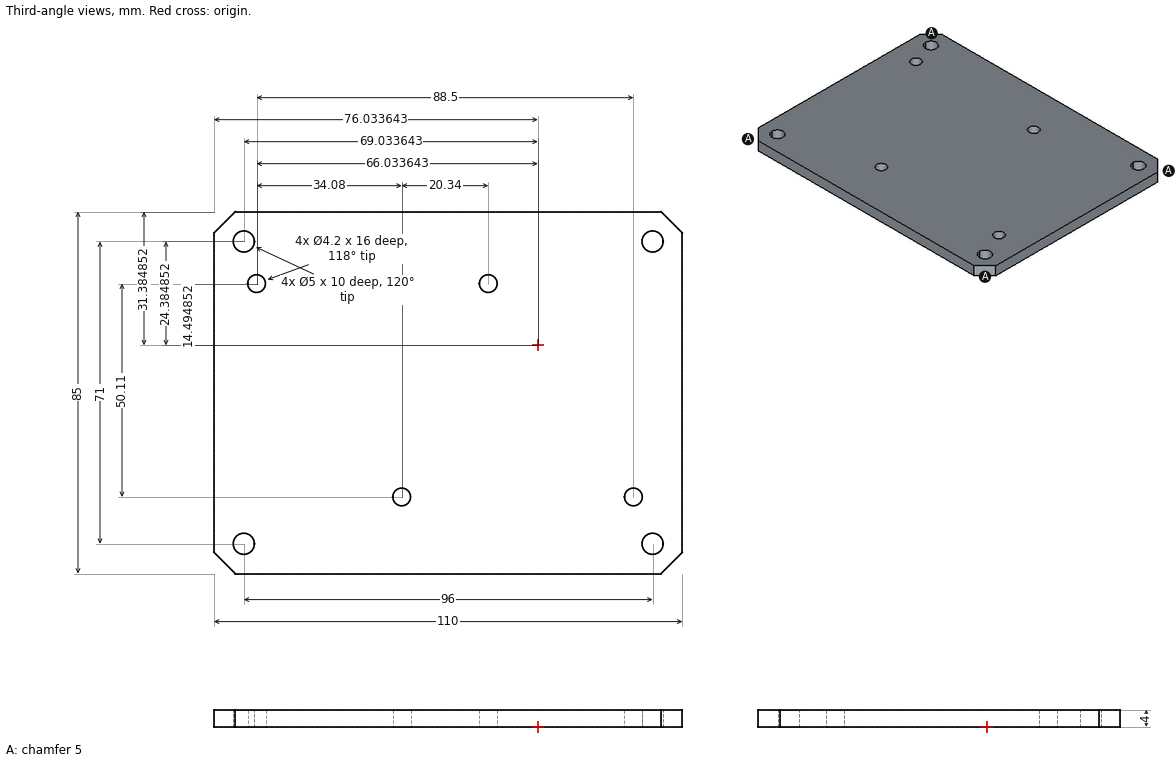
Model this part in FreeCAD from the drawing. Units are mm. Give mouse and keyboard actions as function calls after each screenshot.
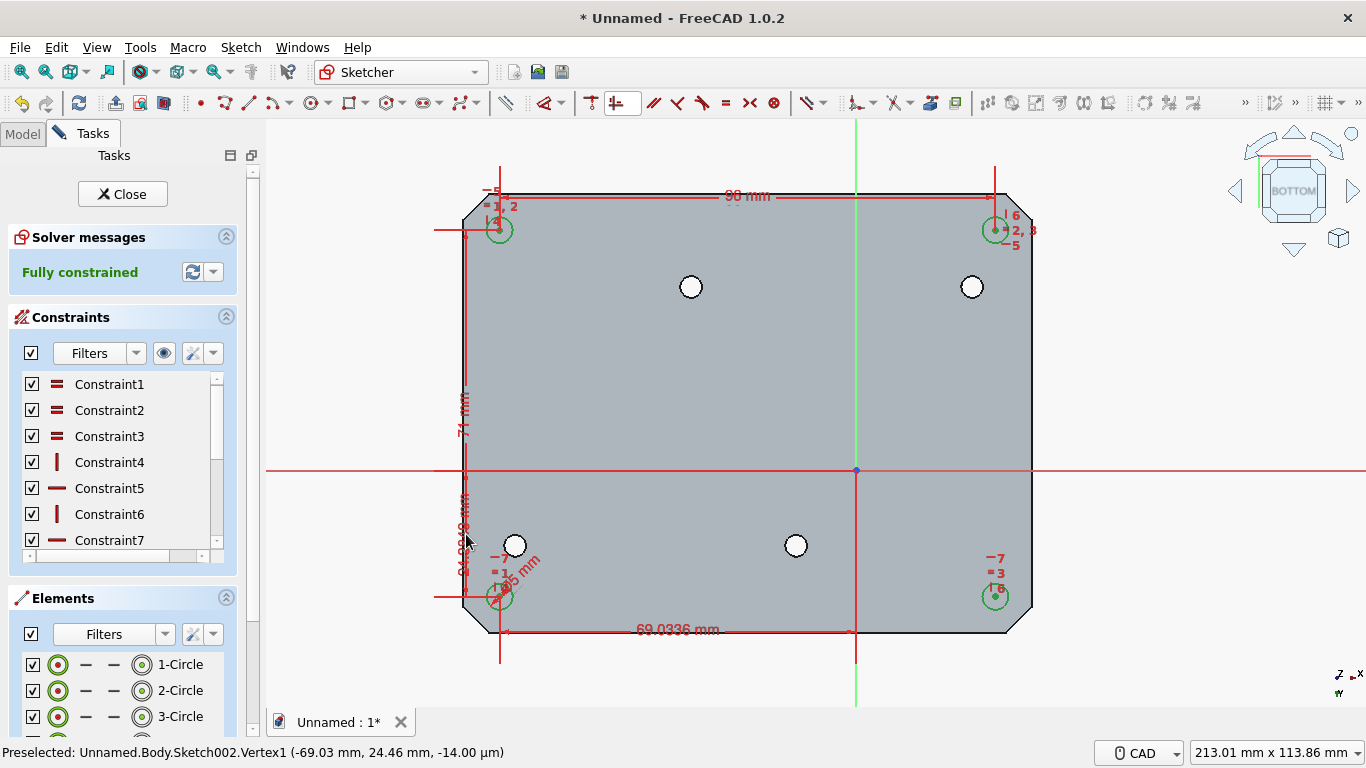
click(123, 194)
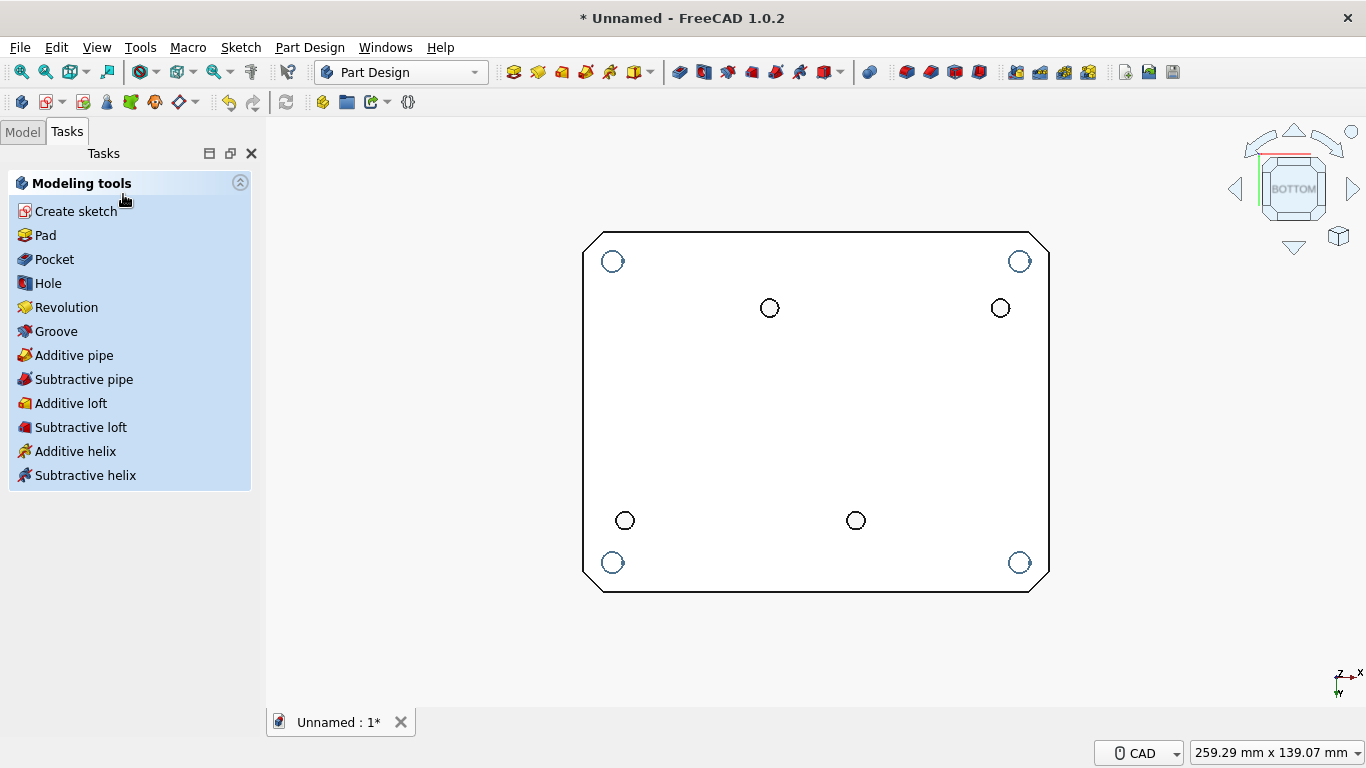
click(704, 72)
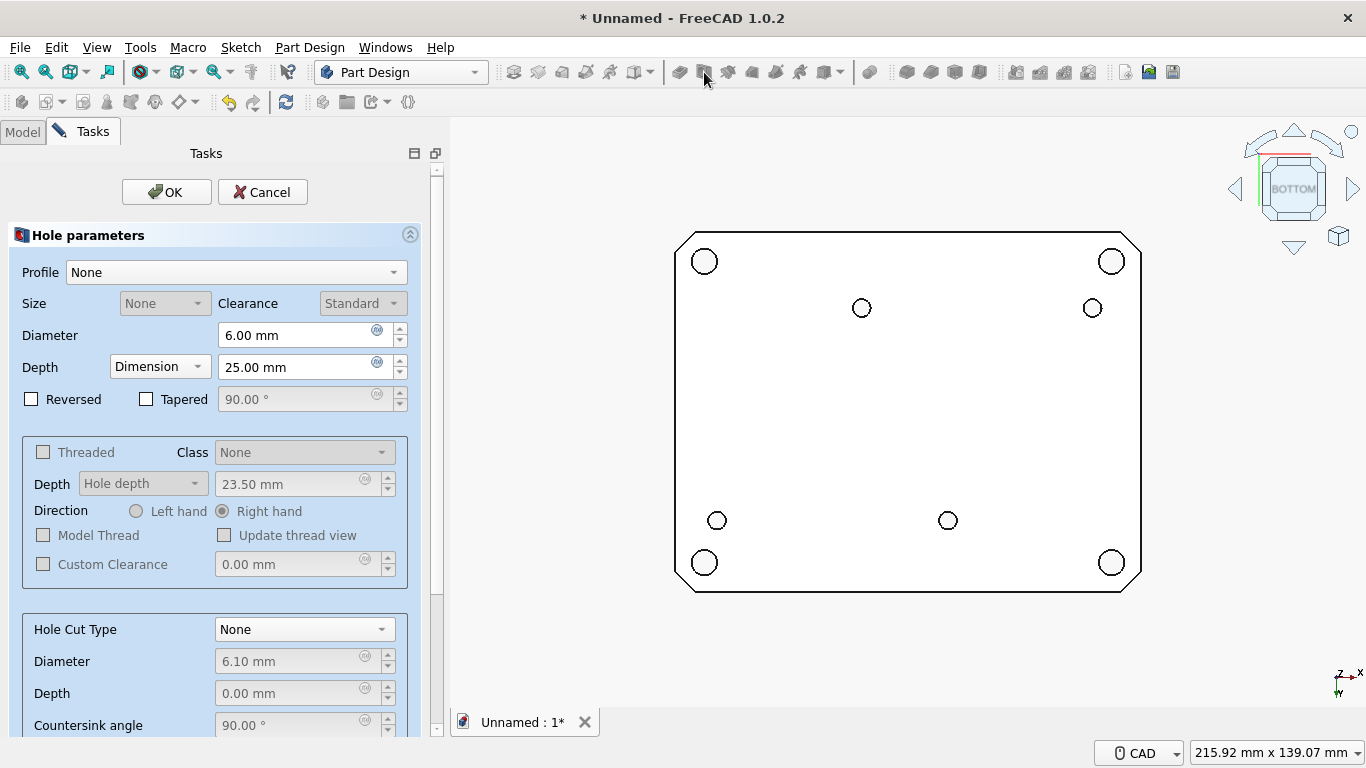
triple_click(305, 335)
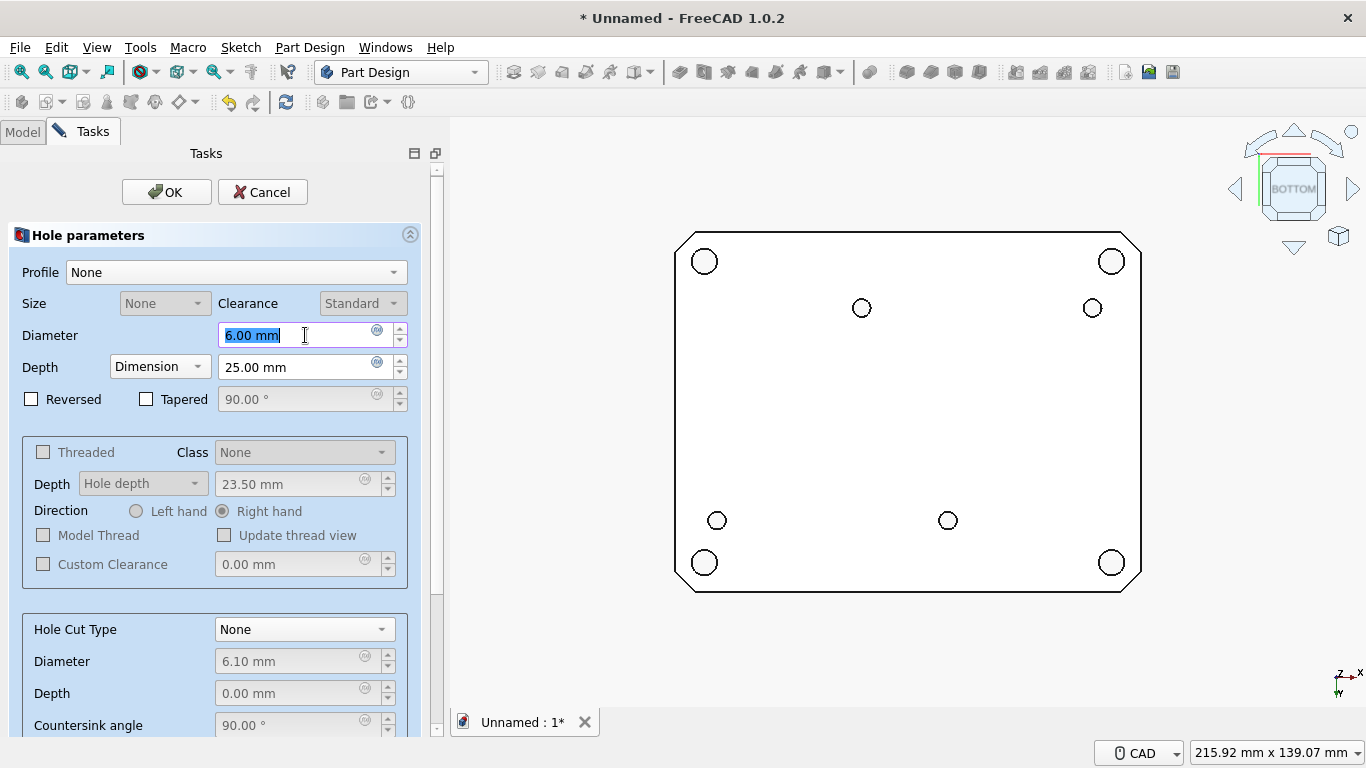
text(5)
key(Tab)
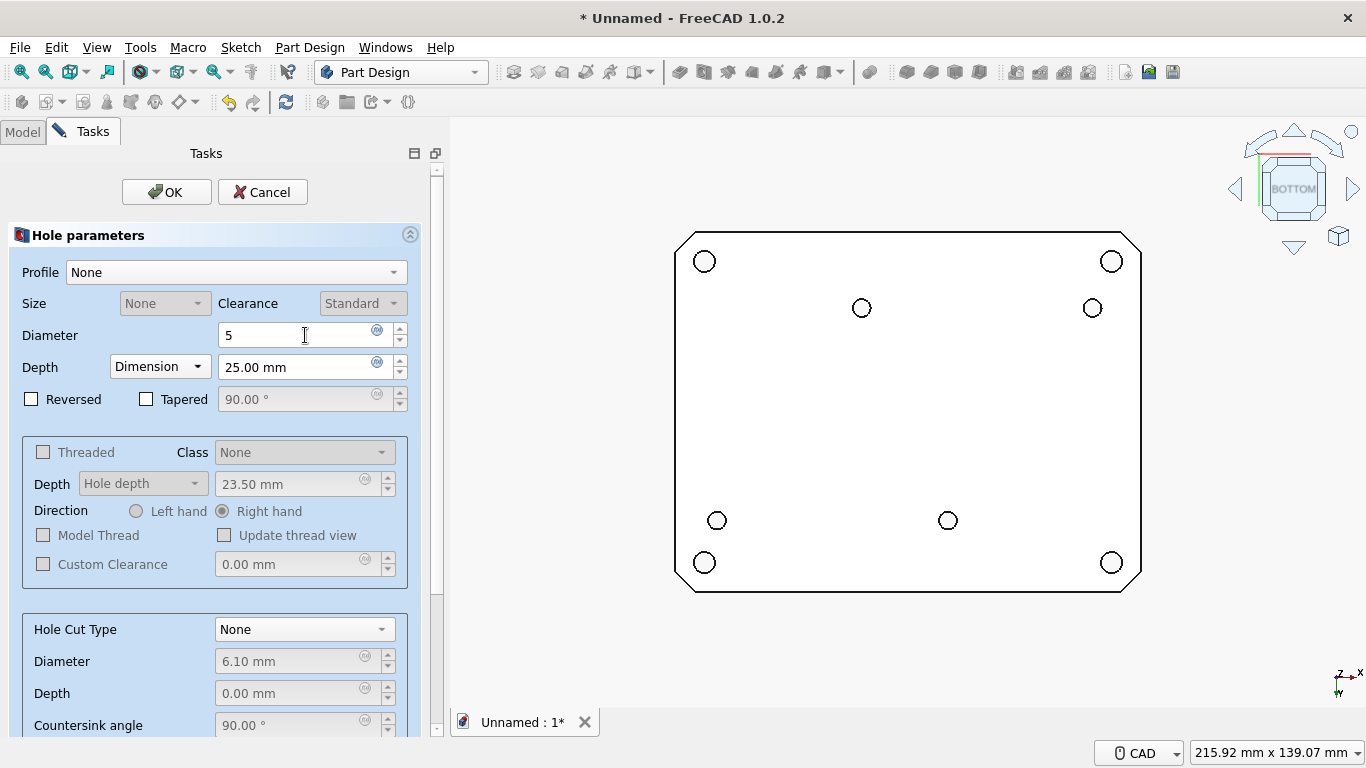
triple_click(305, 367)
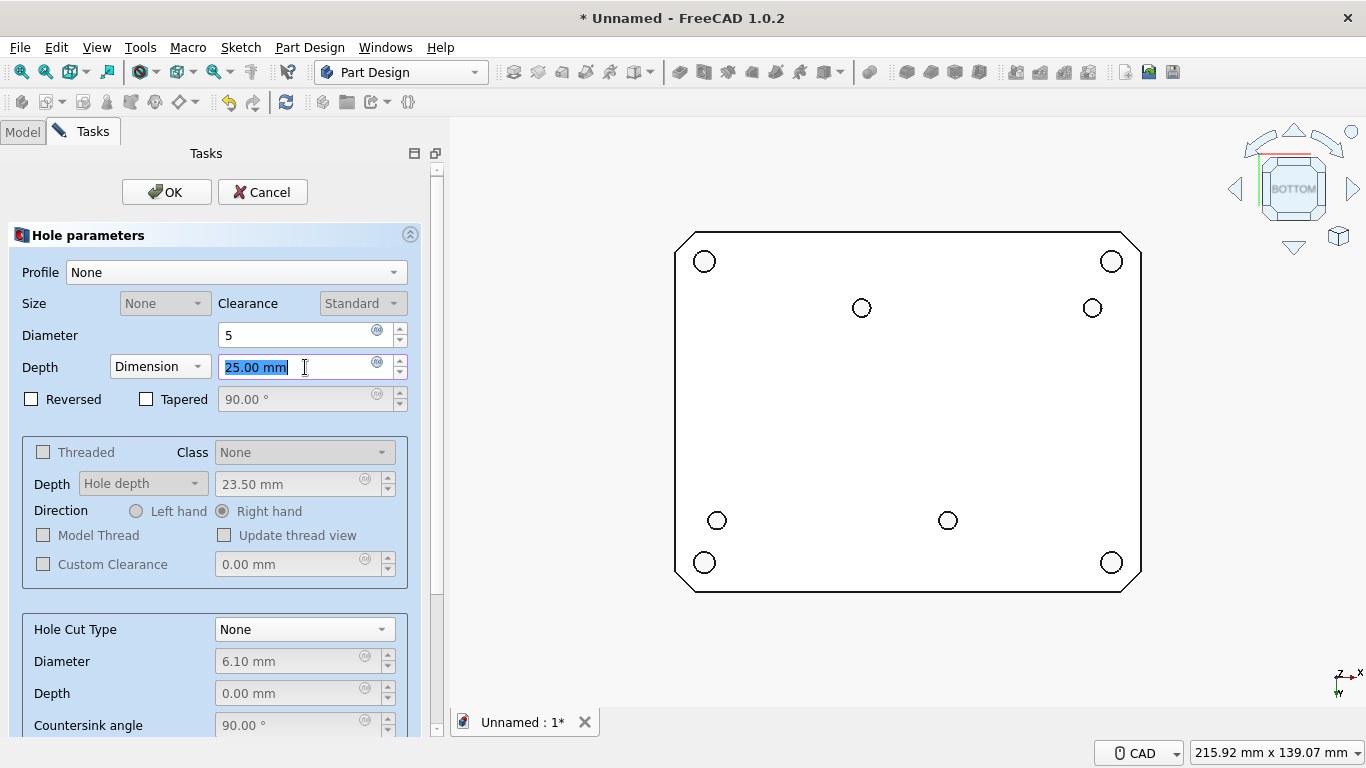
text(10)
key(Tab)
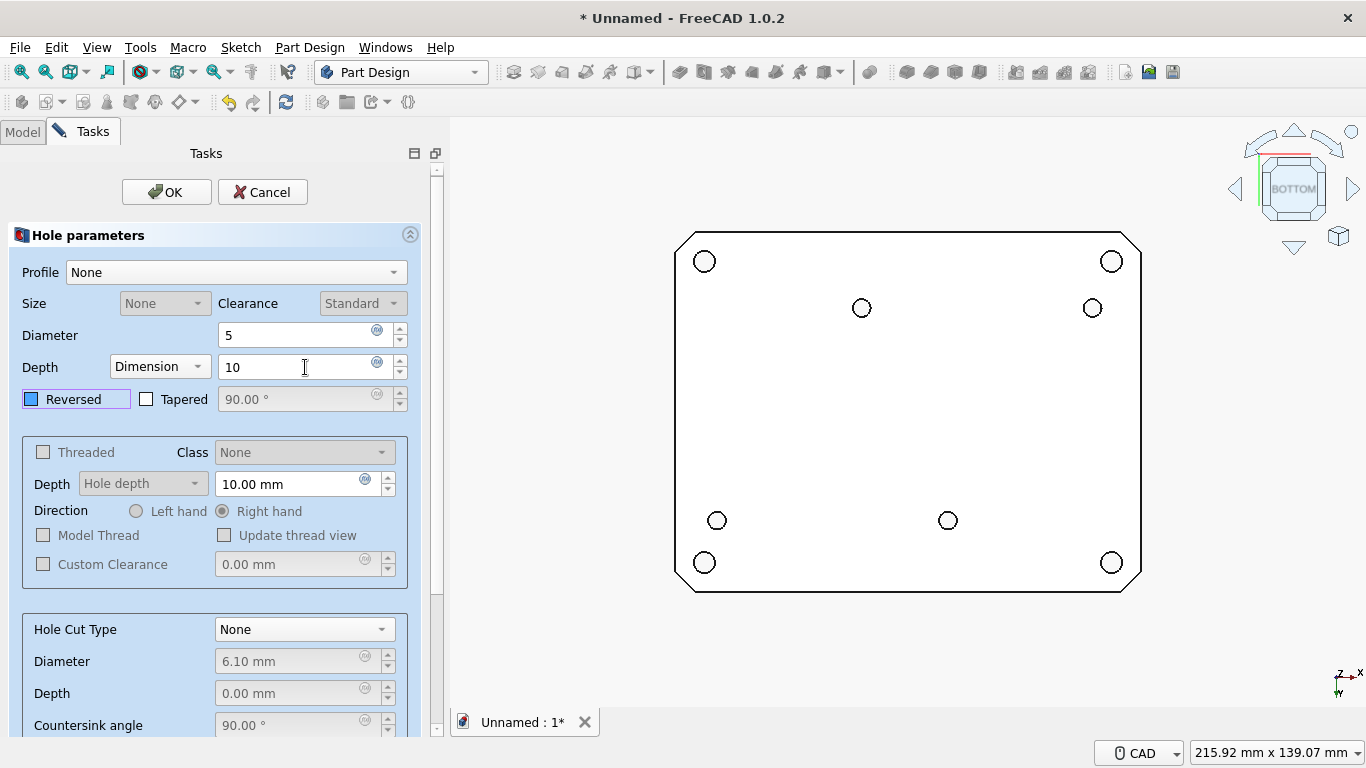
scroll(437, 450, down, 3)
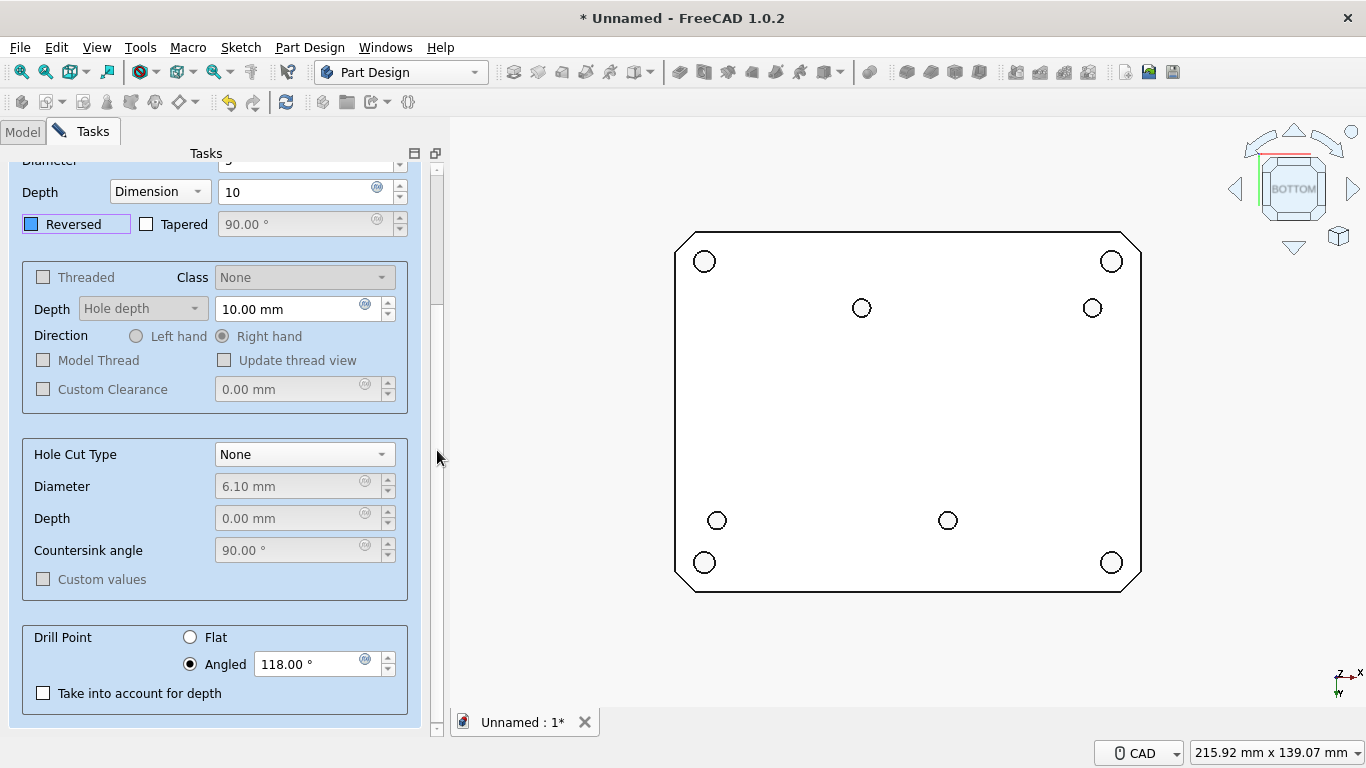
triple_click(317, 664)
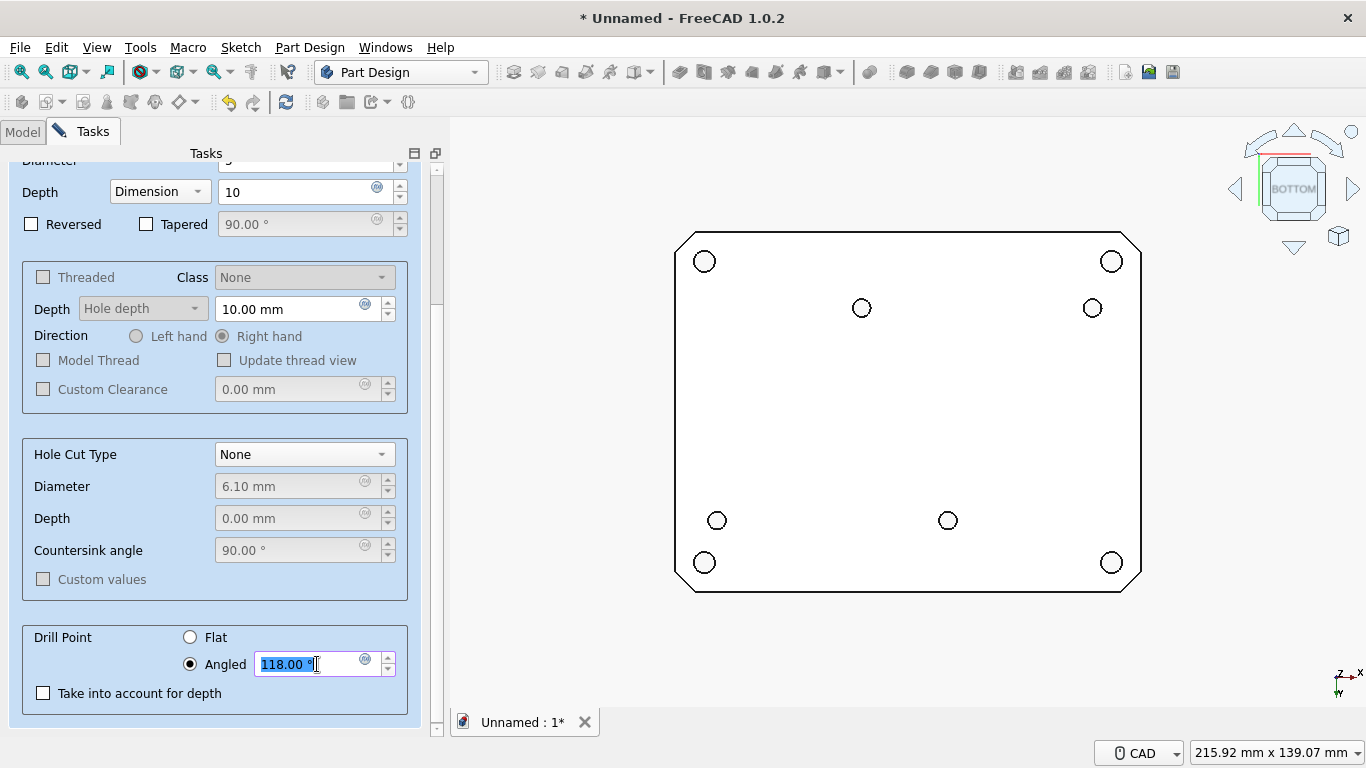
text(120)
key(Tab)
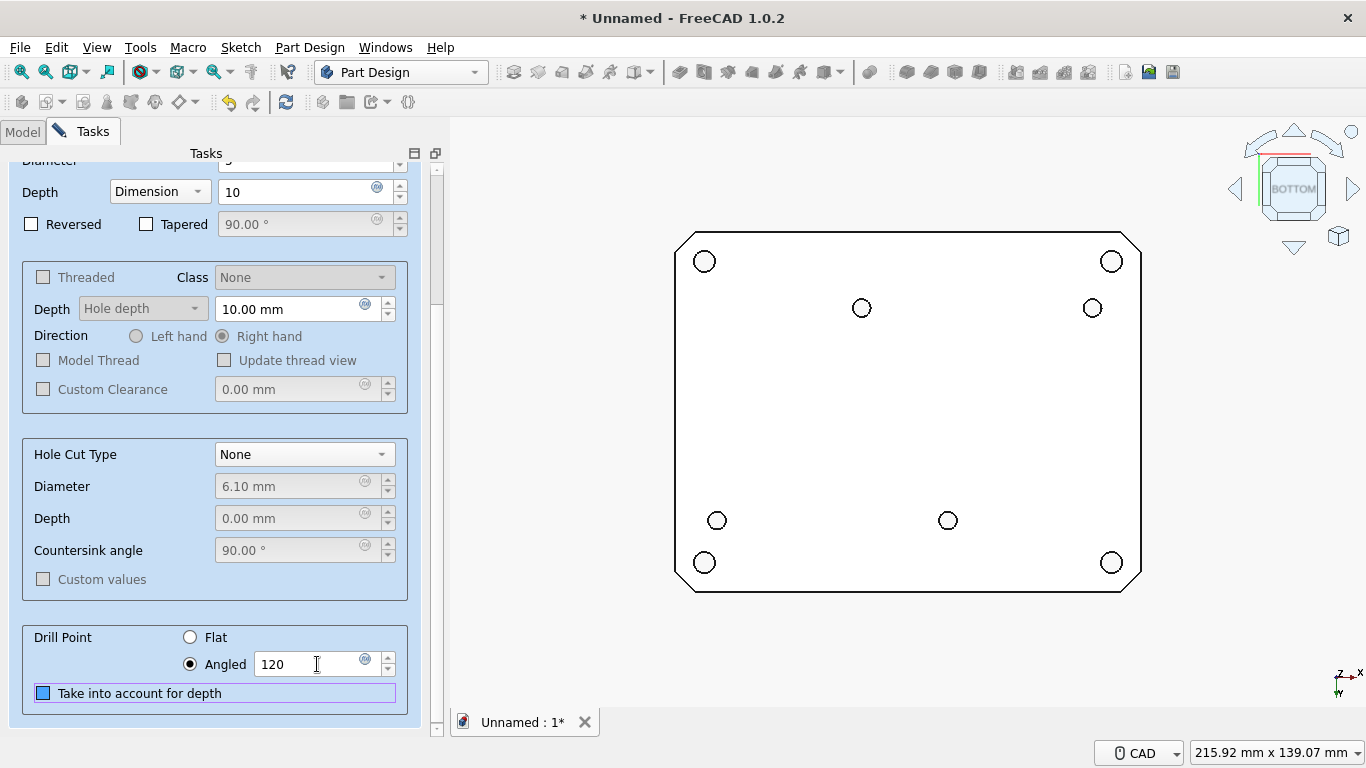
scroll(437, 450, up, 4)